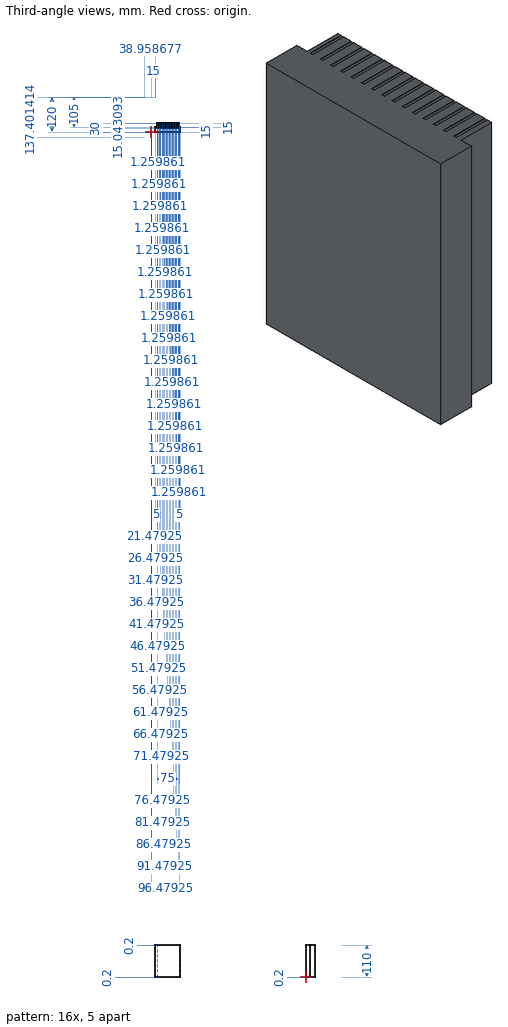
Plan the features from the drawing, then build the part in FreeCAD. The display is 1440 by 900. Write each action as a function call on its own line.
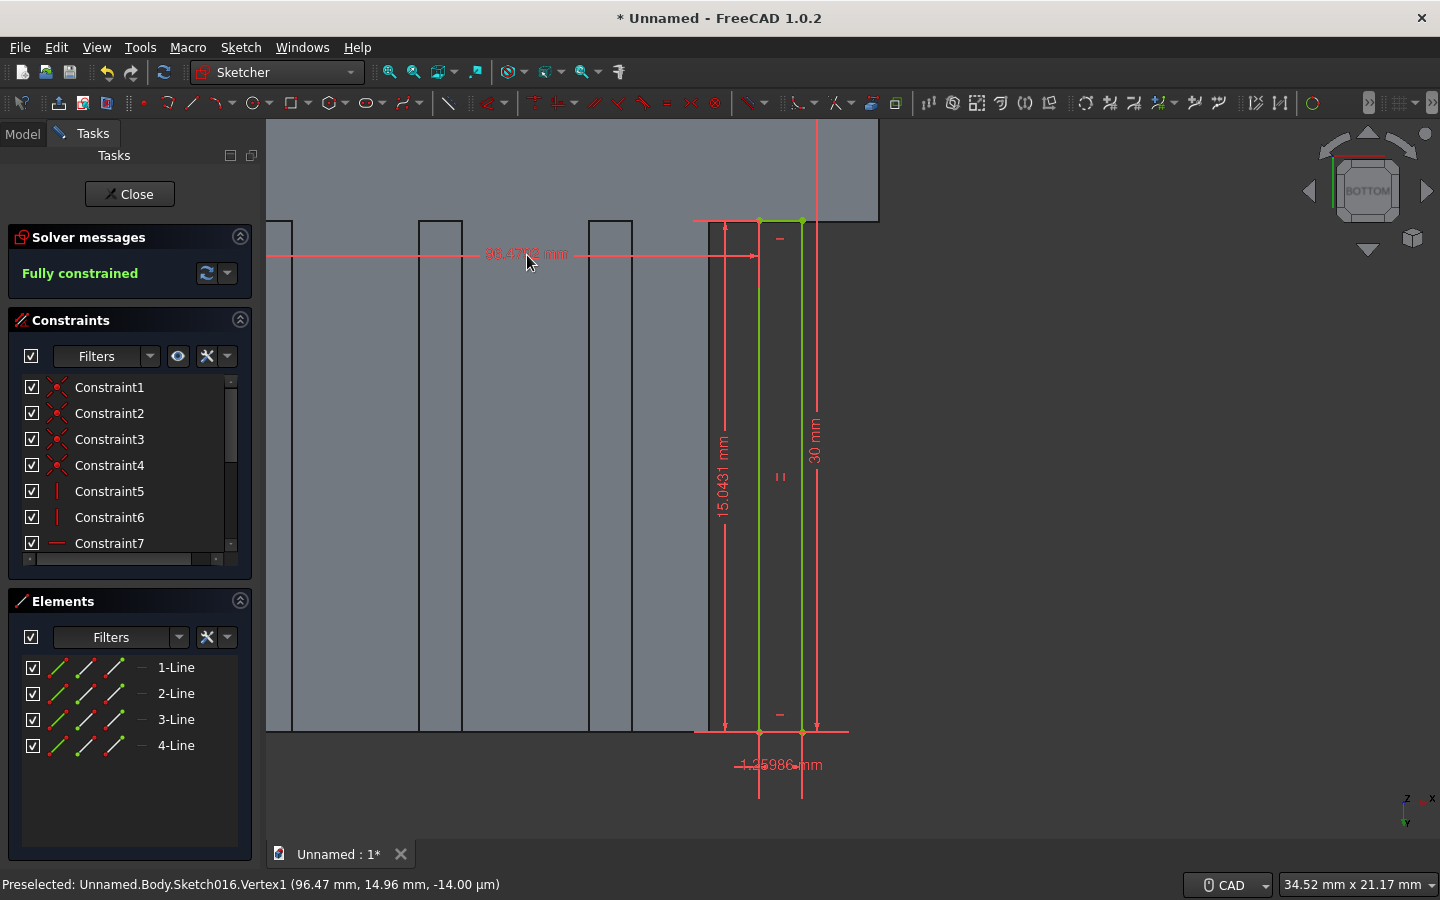
click(130, 194)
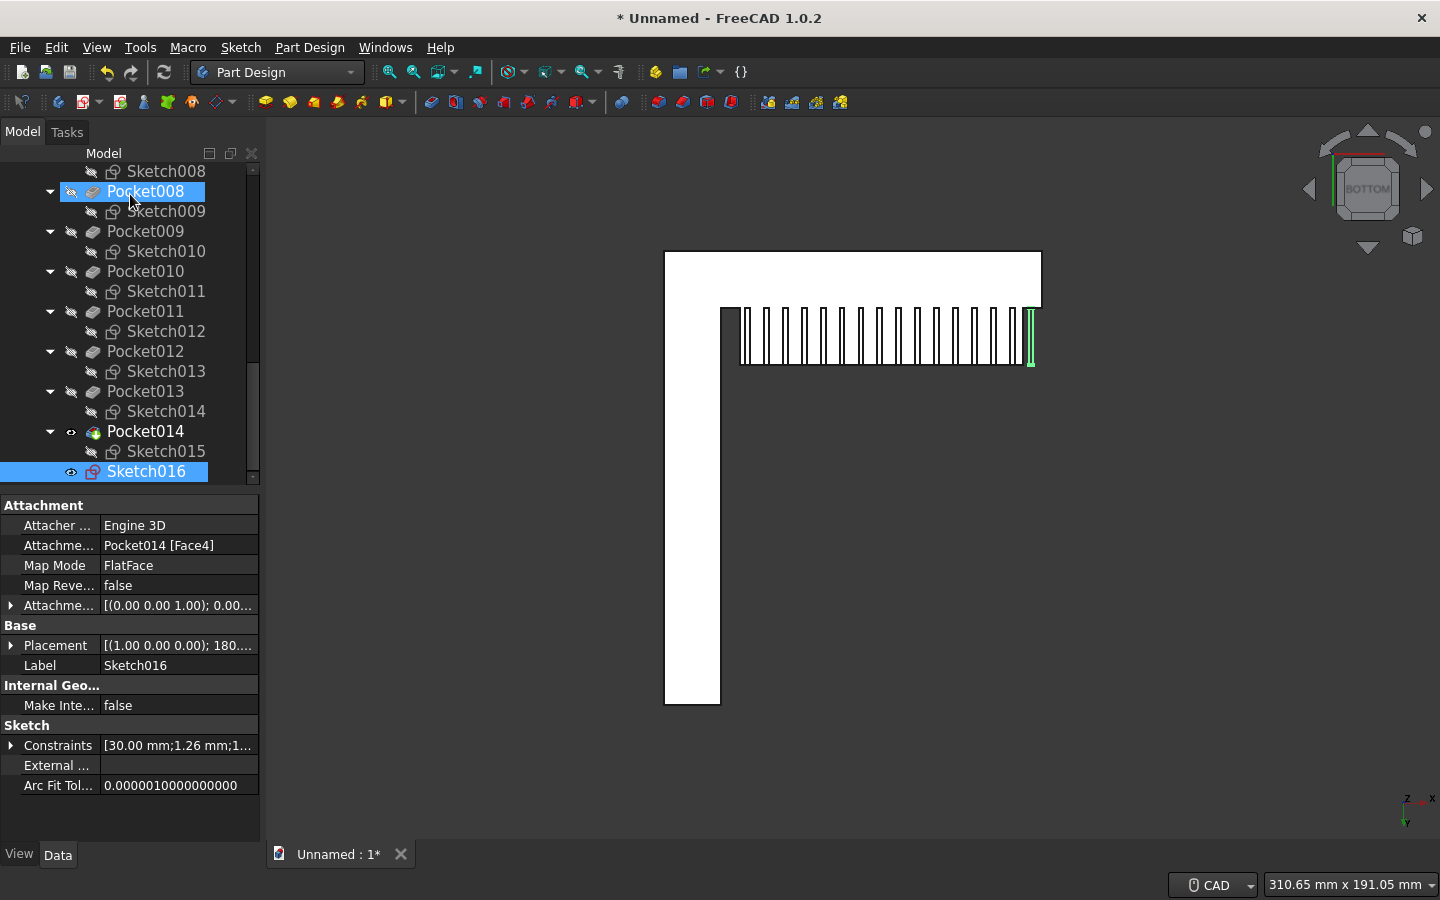
click(432, 102)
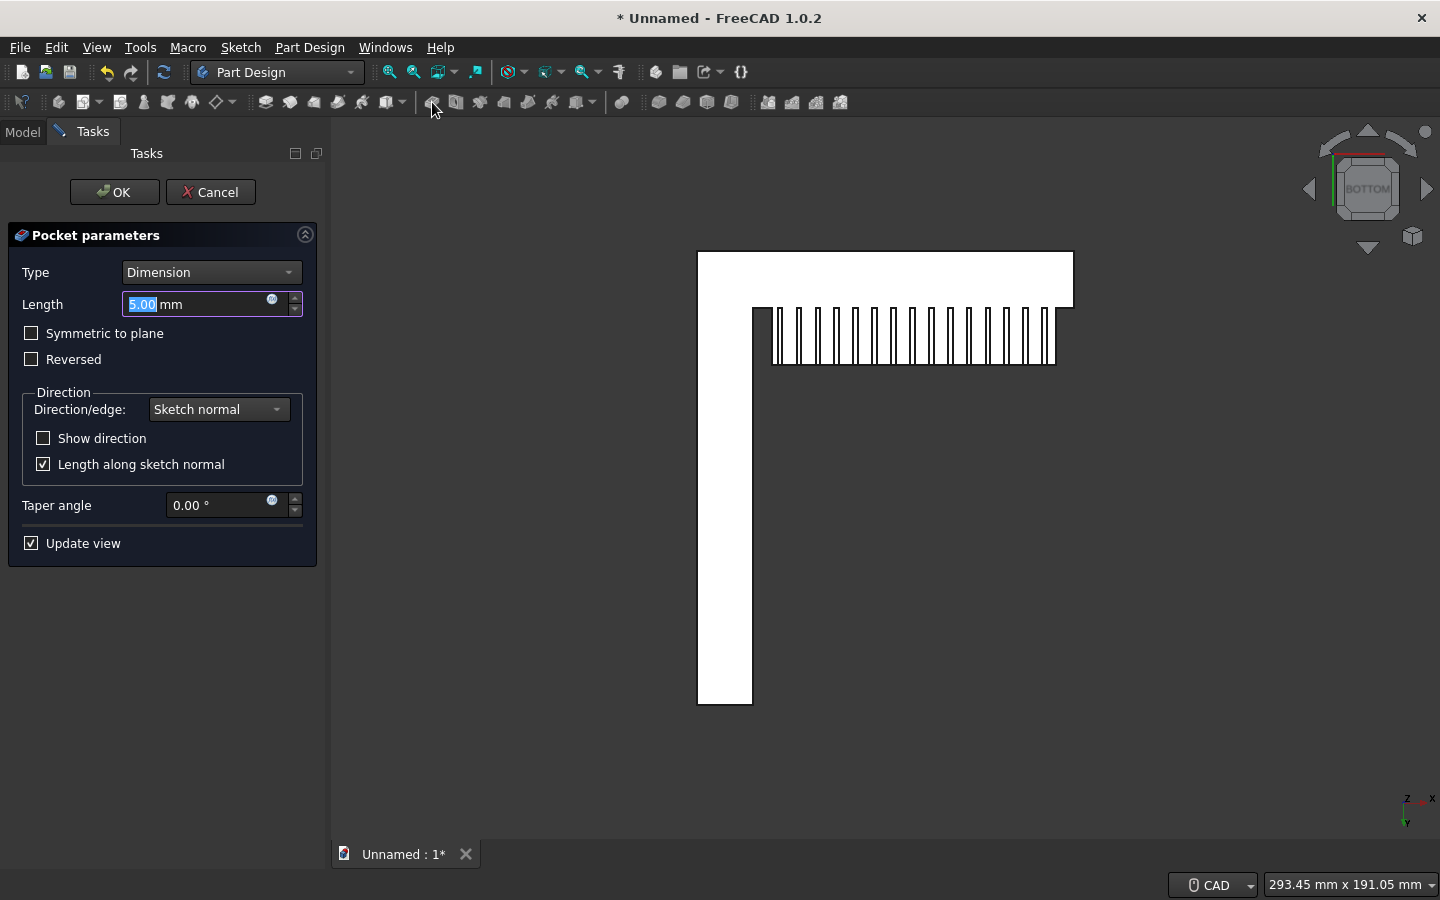
text(0.2)
key(Tab)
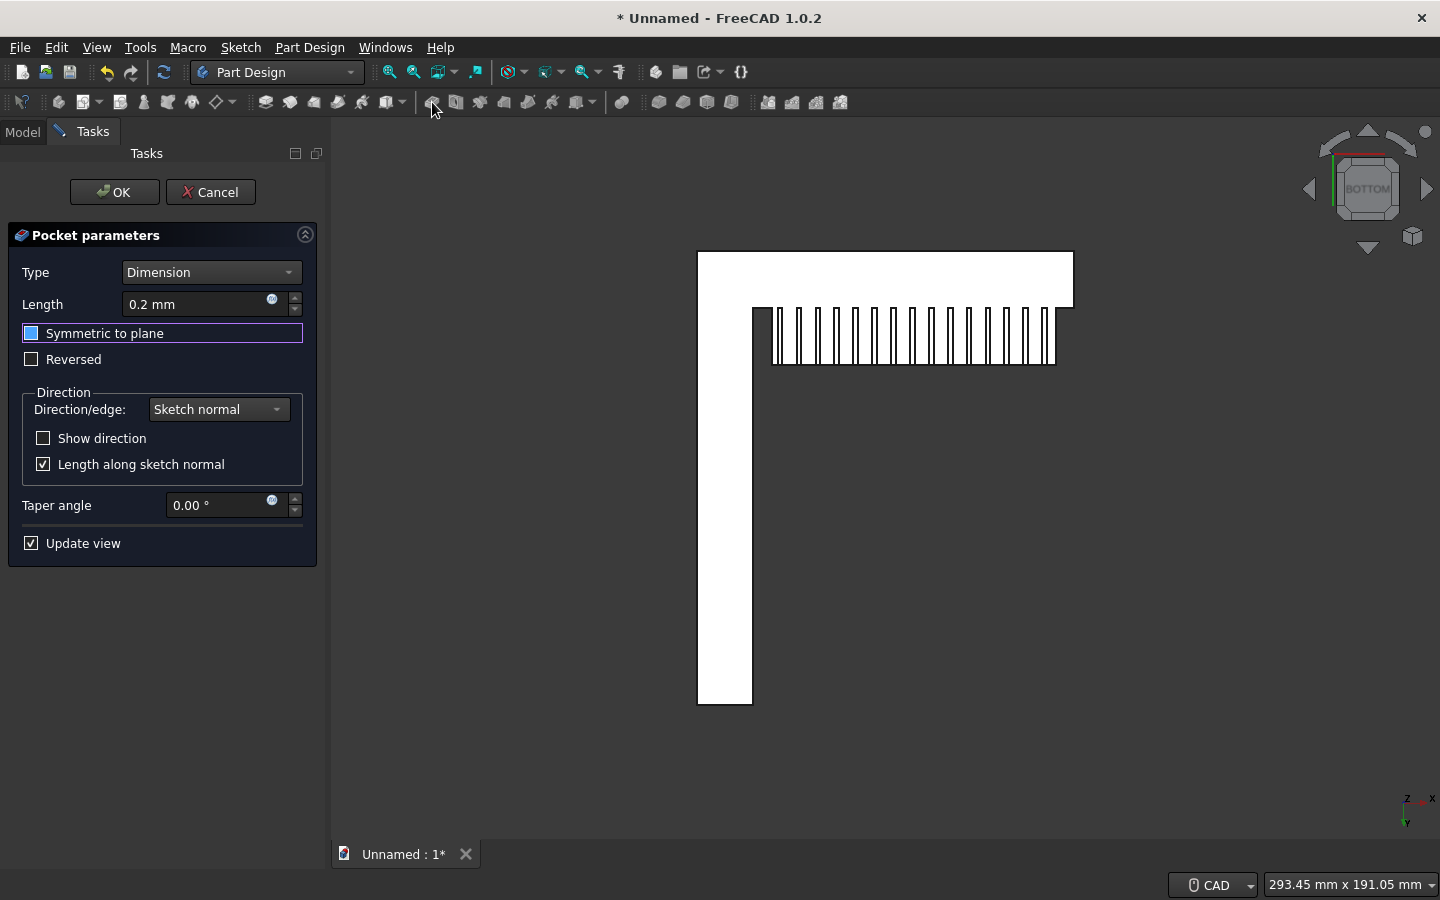
click(115, 192)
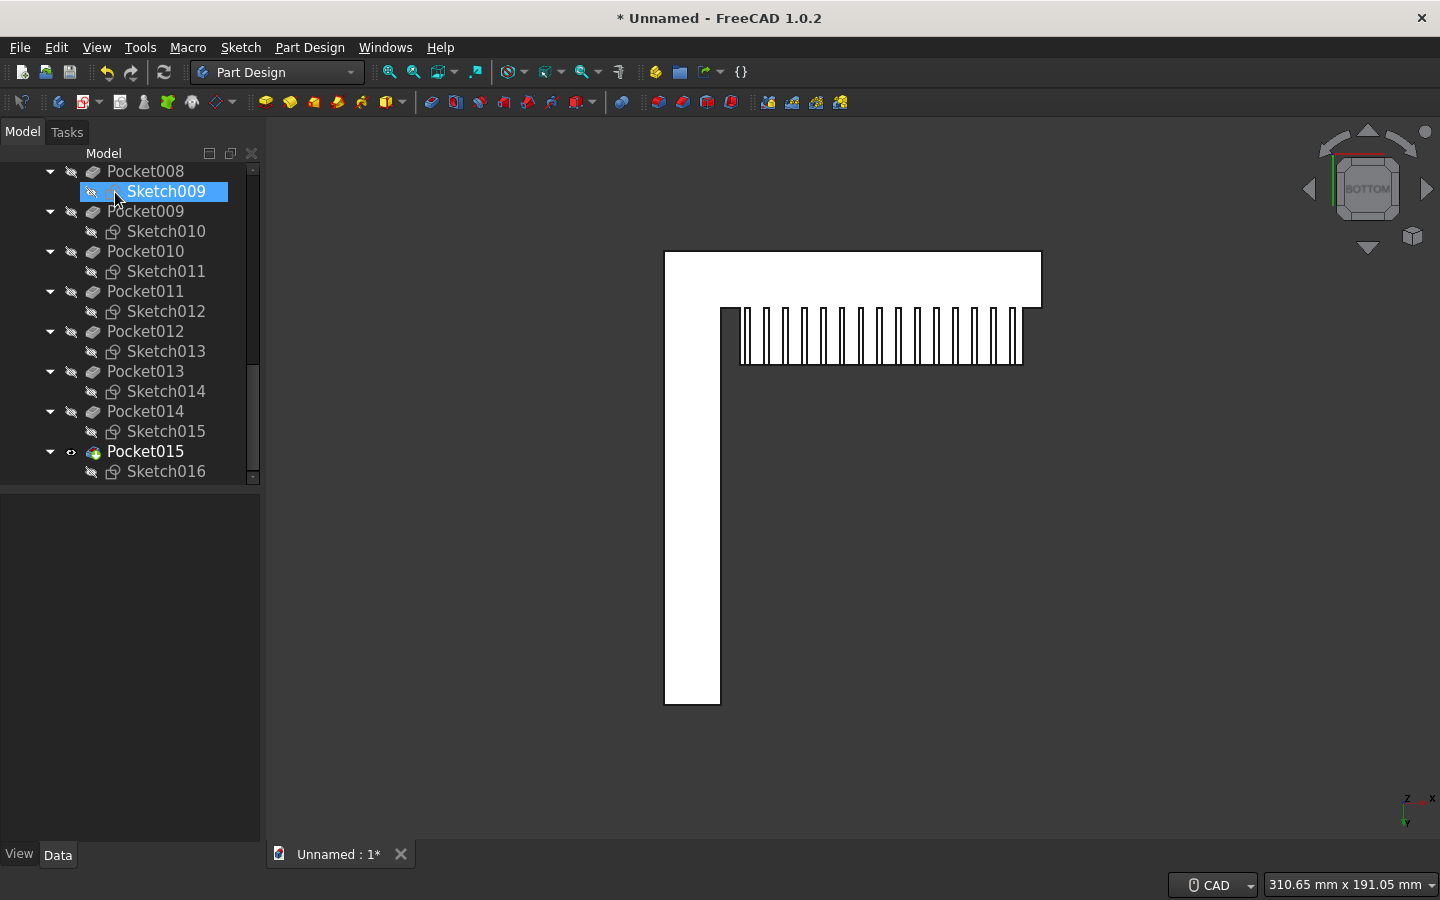
click(691, 671)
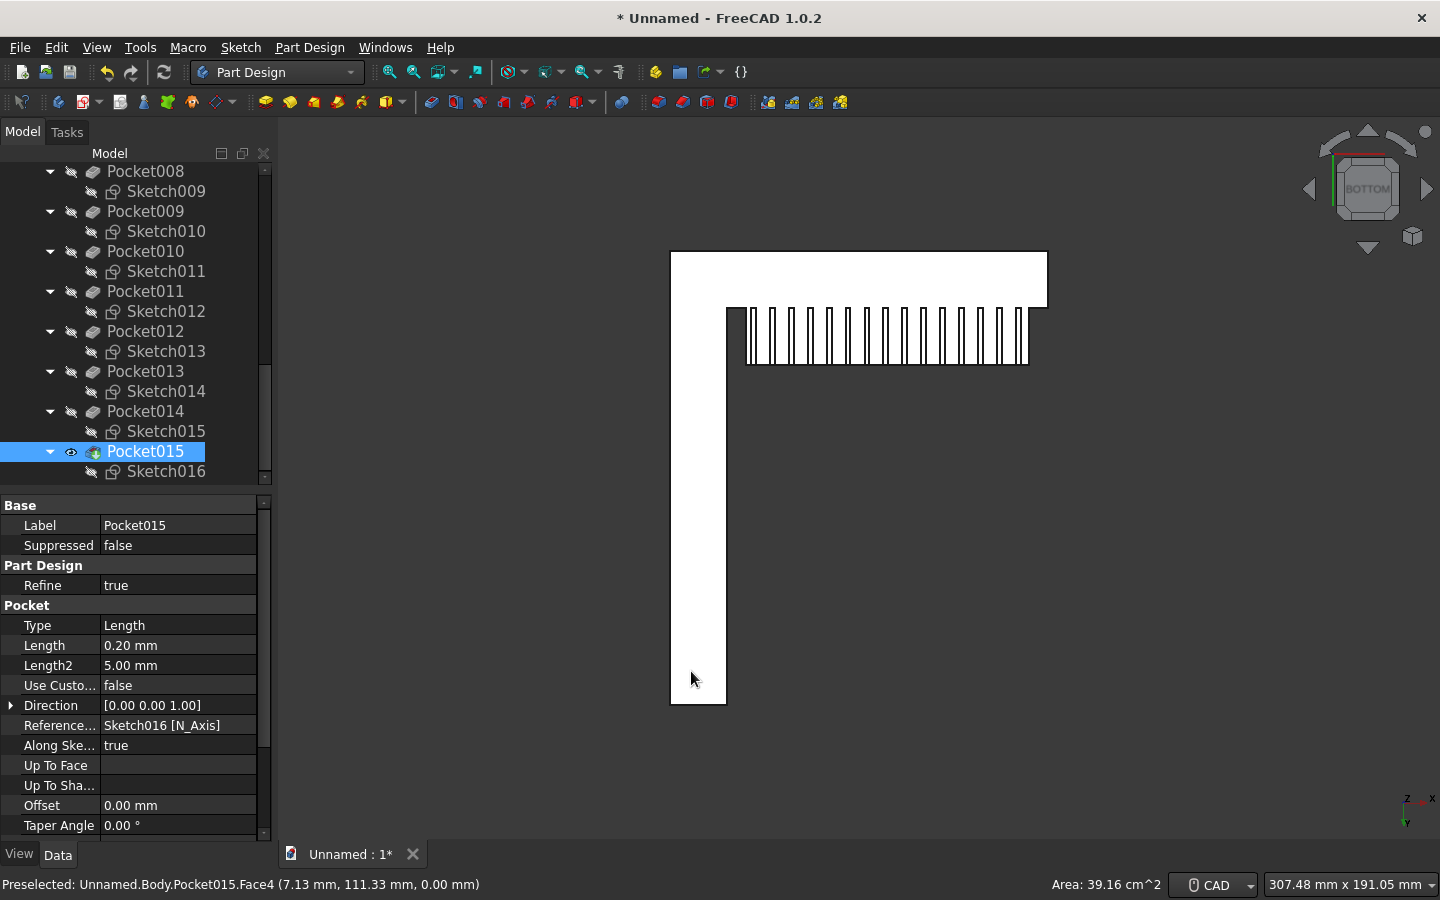
click(84, 102)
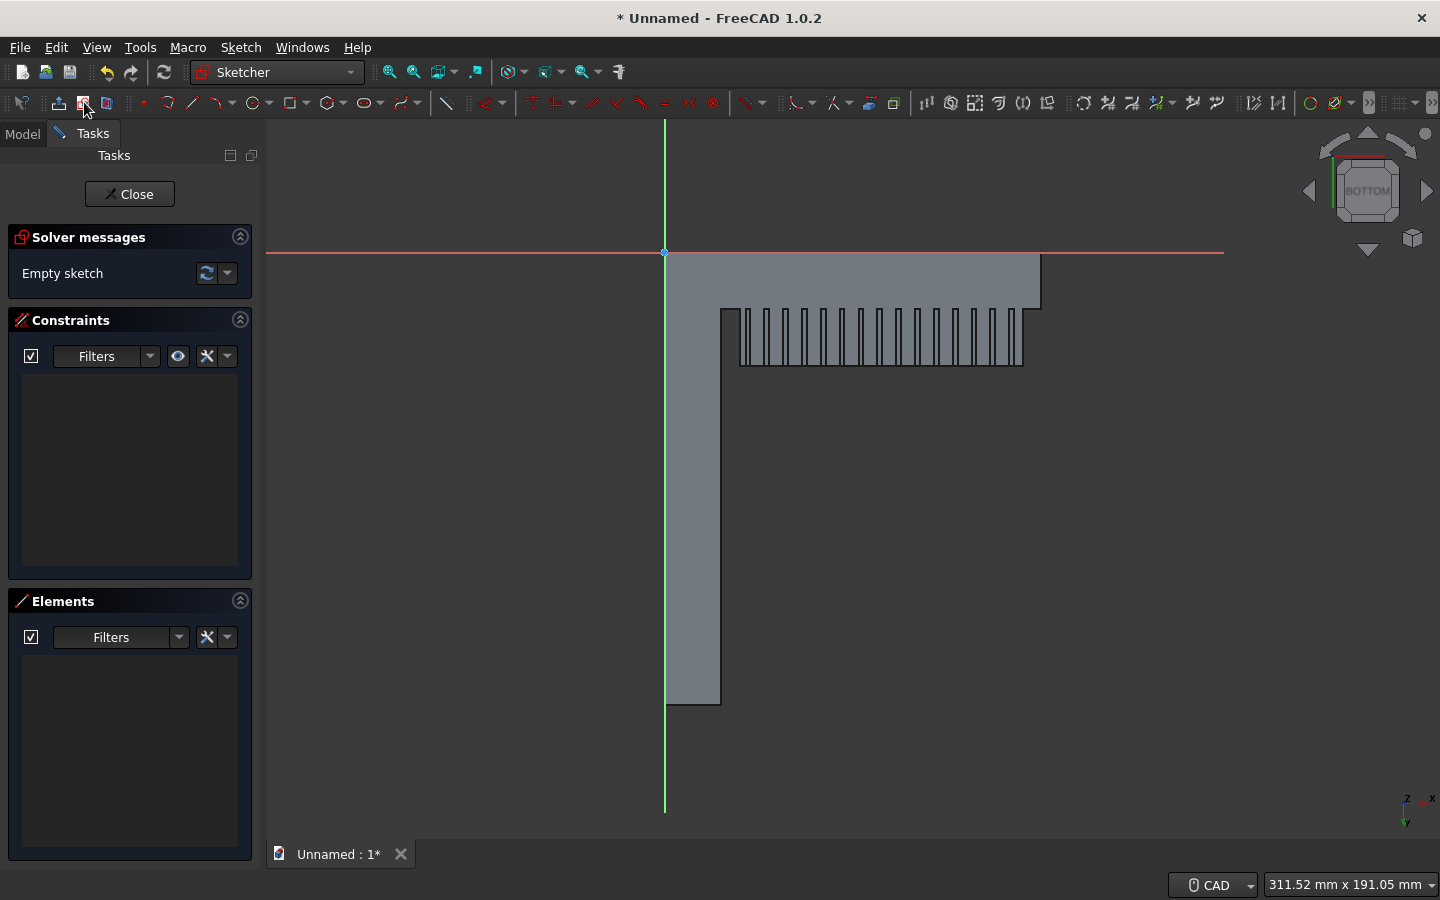
key(g)
key(r)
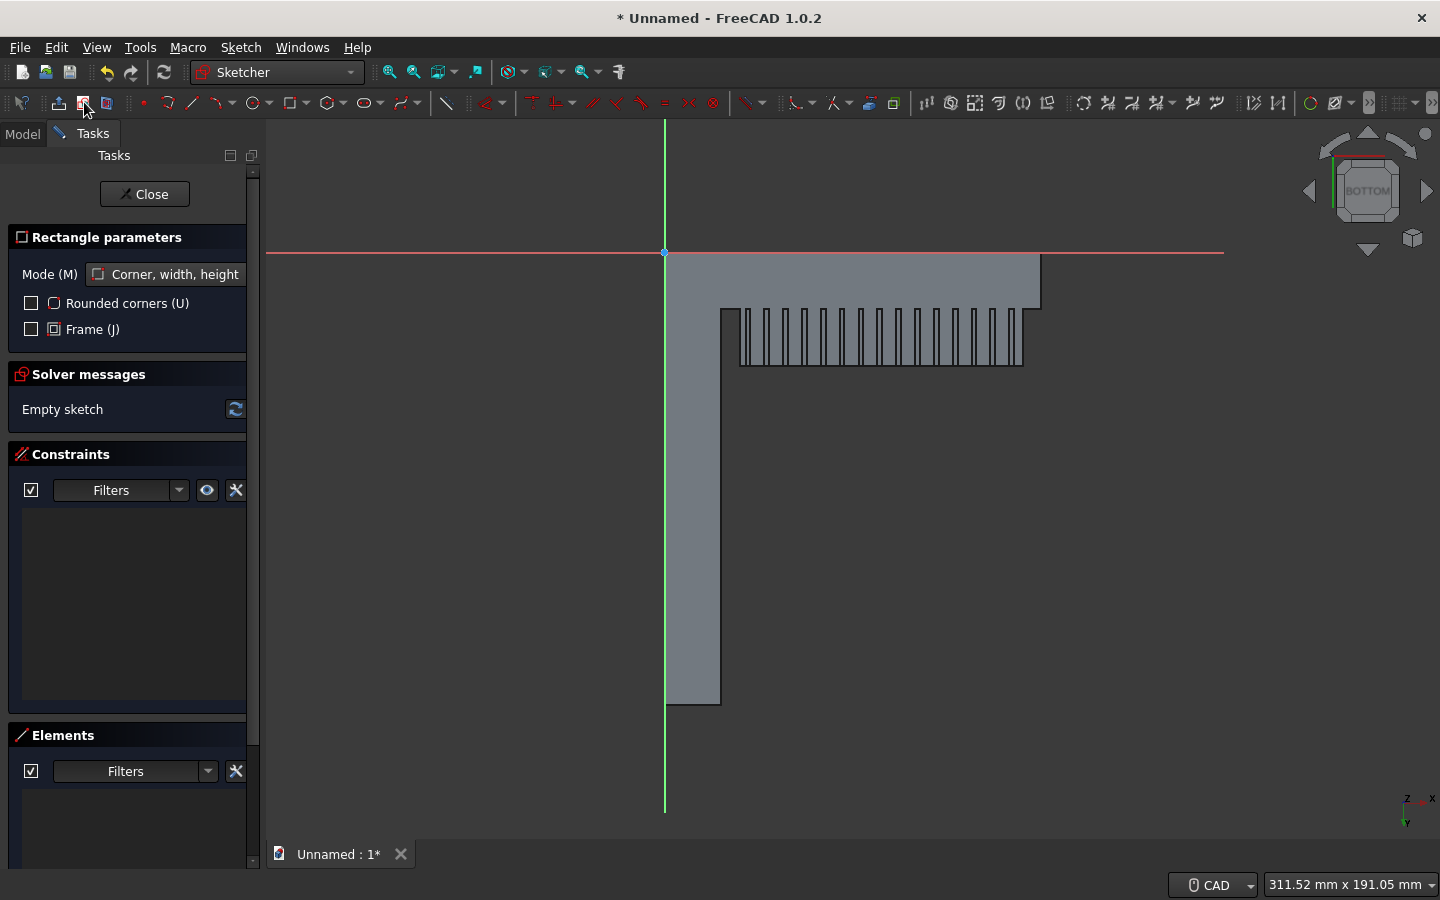
click(574, 187)
click(721, 705)
key(Escape)